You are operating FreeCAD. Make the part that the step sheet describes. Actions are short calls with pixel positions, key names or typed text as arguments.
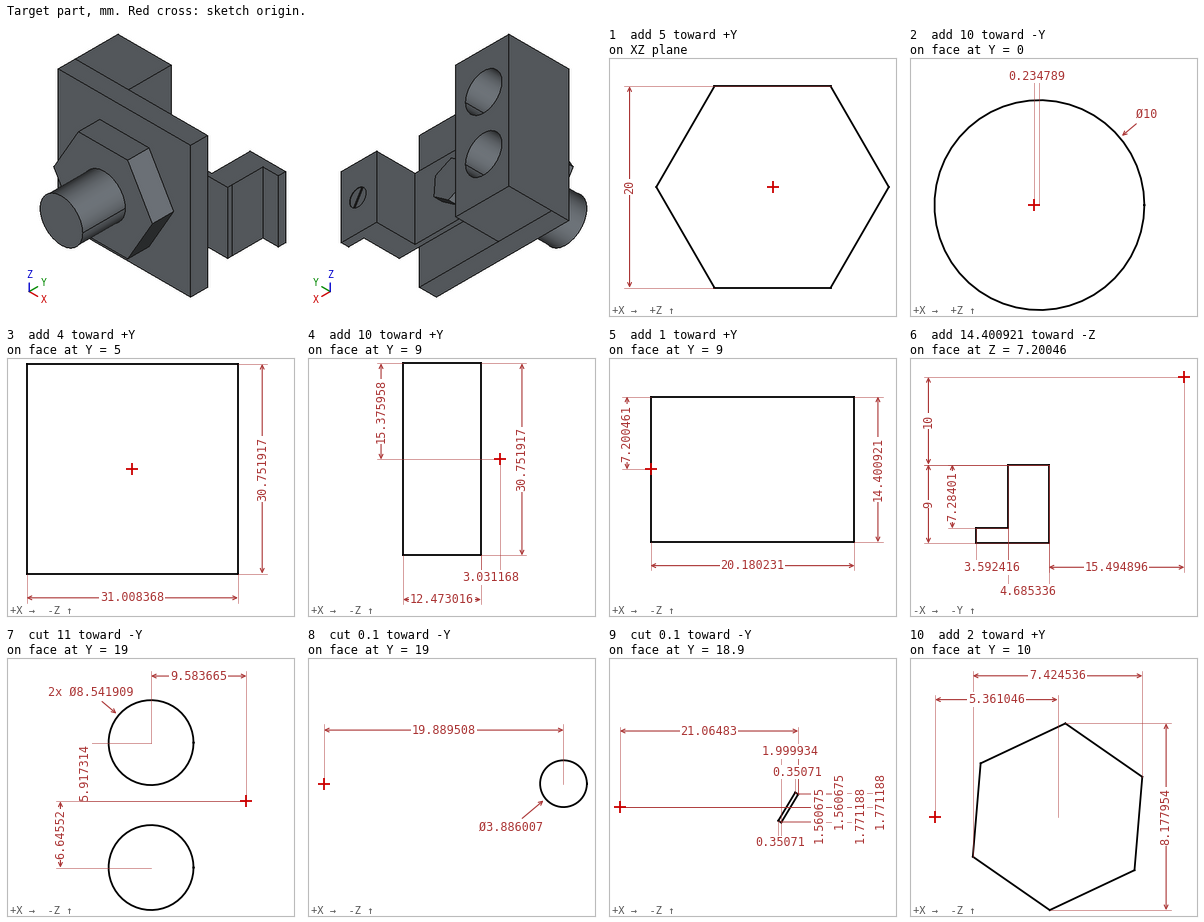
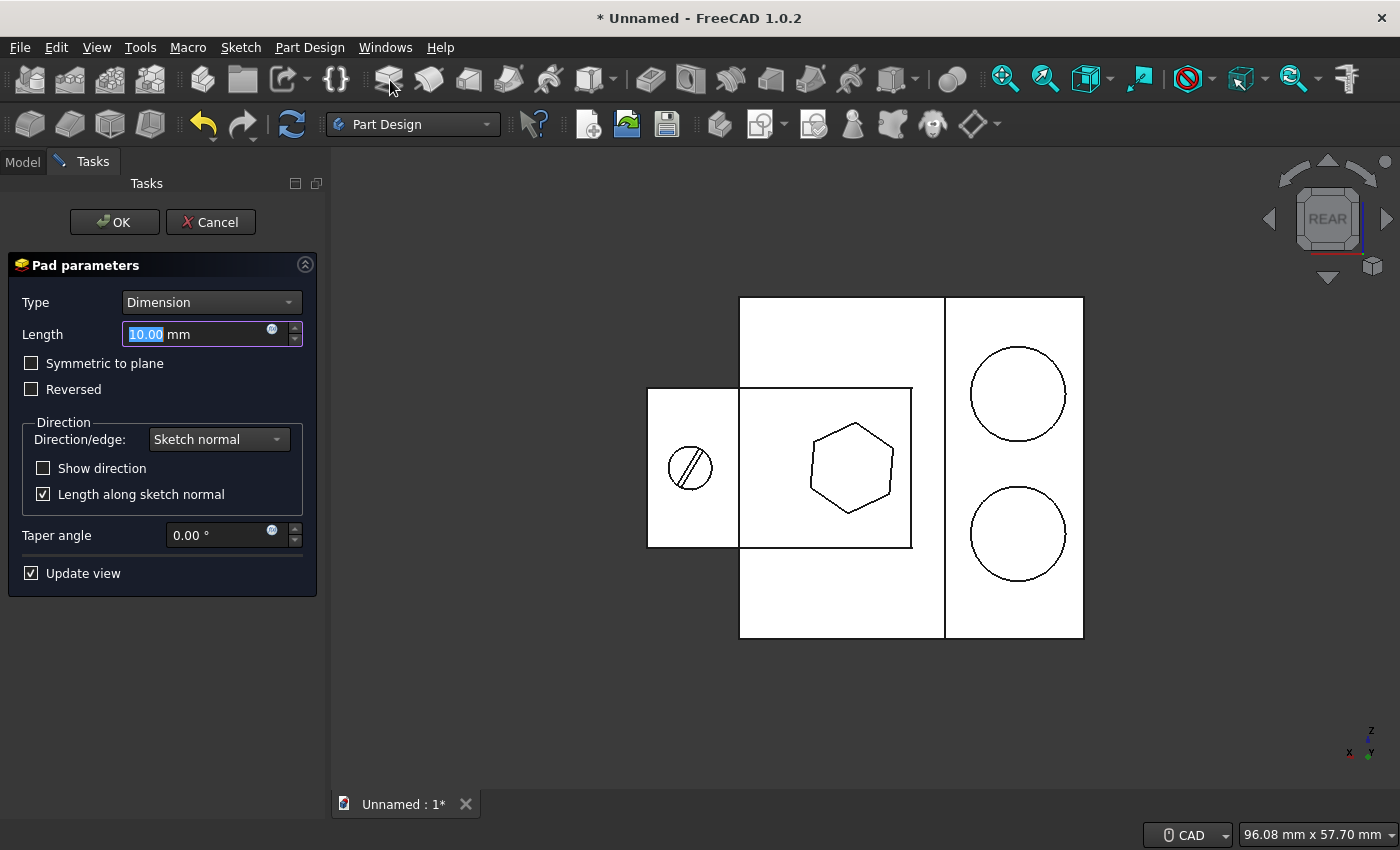
text(2)
key(Tab)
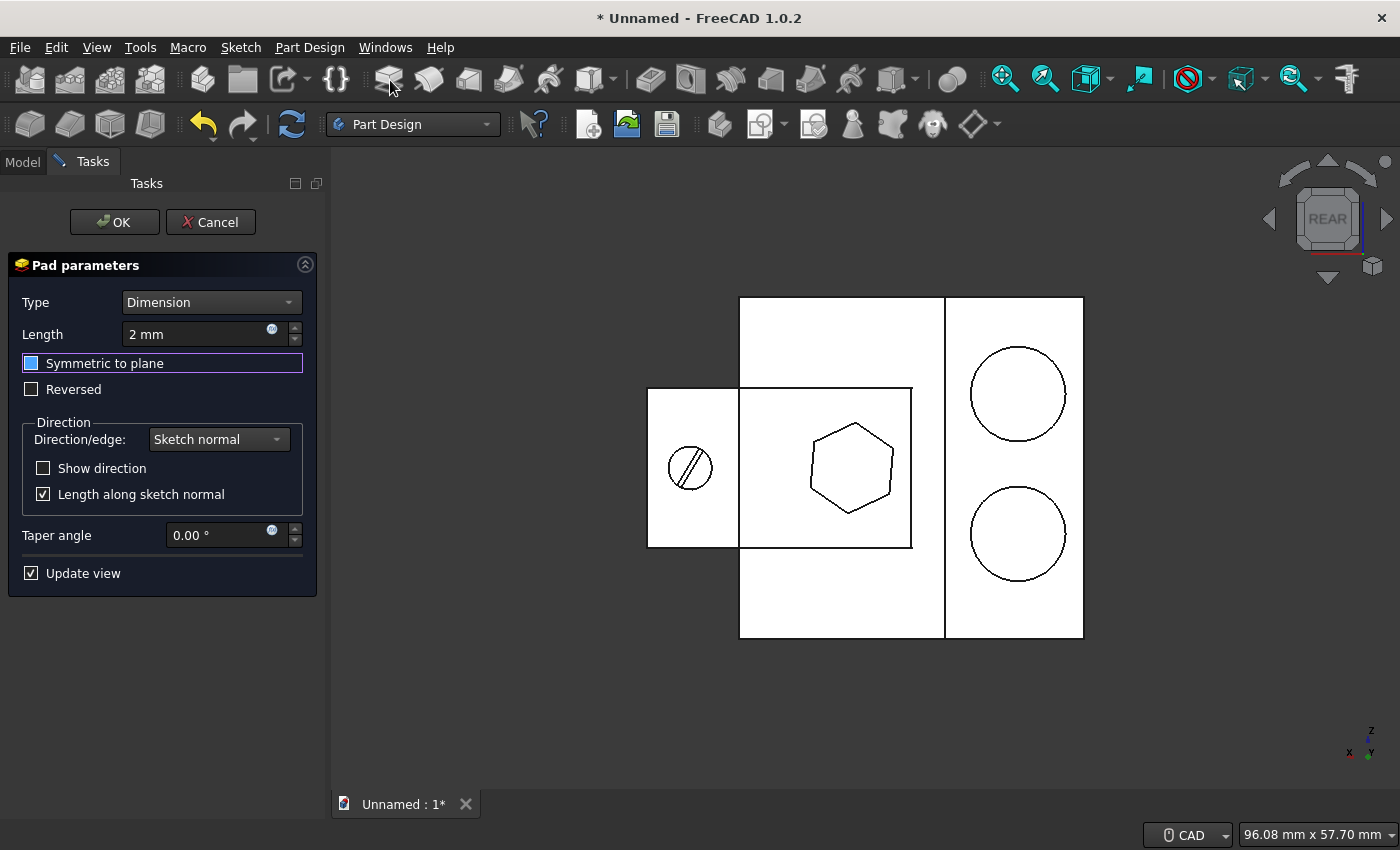
click(115, 222)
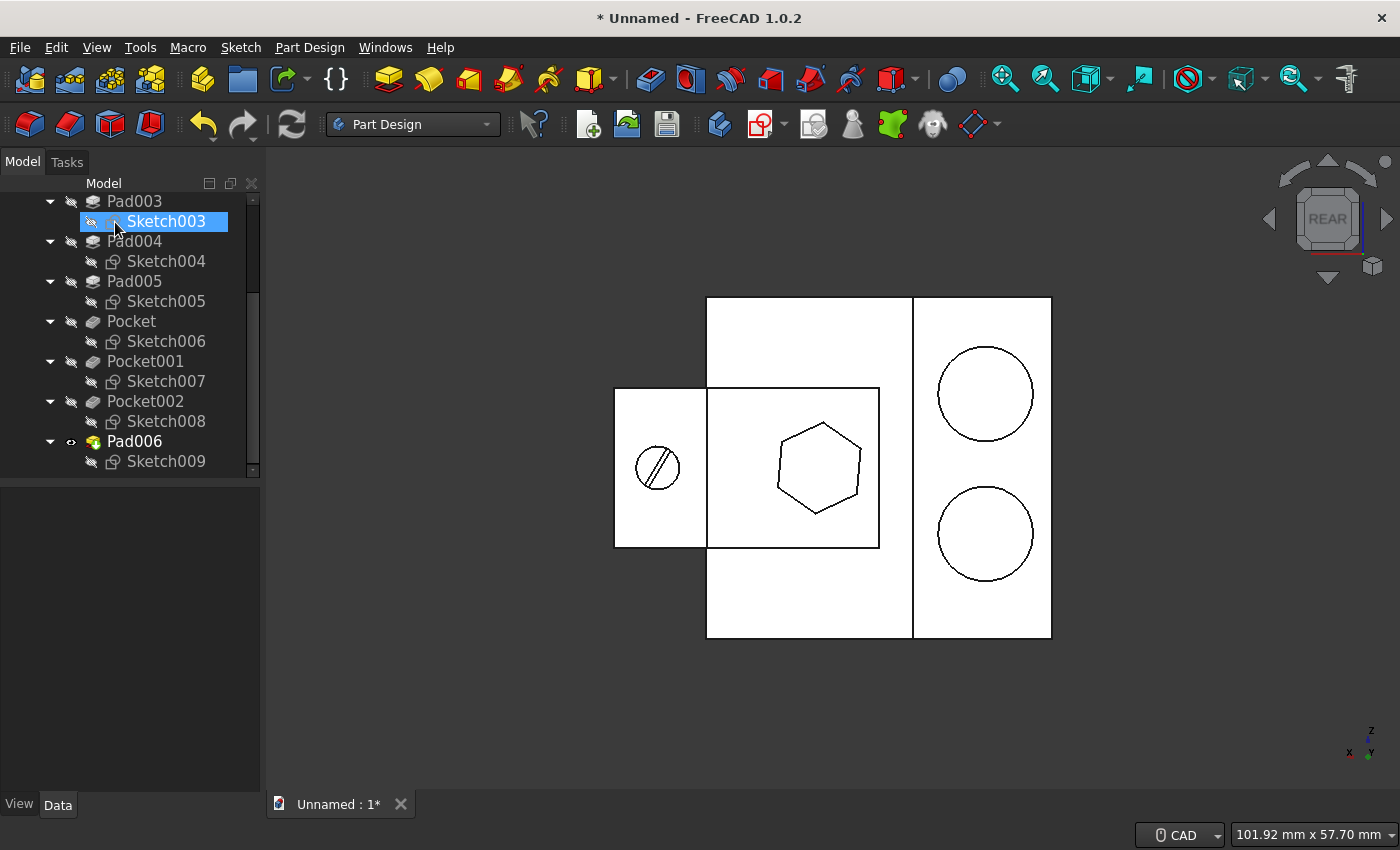
key(0)